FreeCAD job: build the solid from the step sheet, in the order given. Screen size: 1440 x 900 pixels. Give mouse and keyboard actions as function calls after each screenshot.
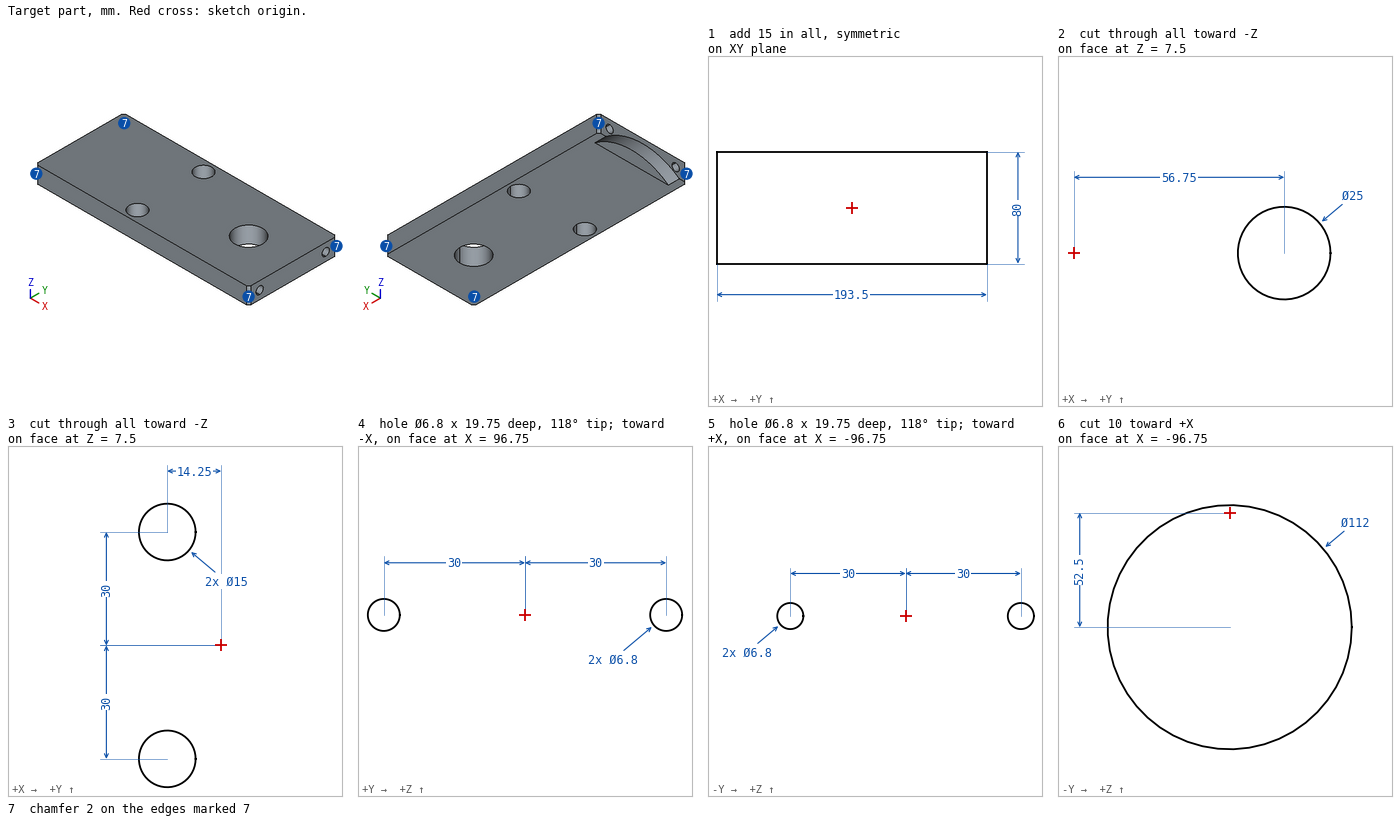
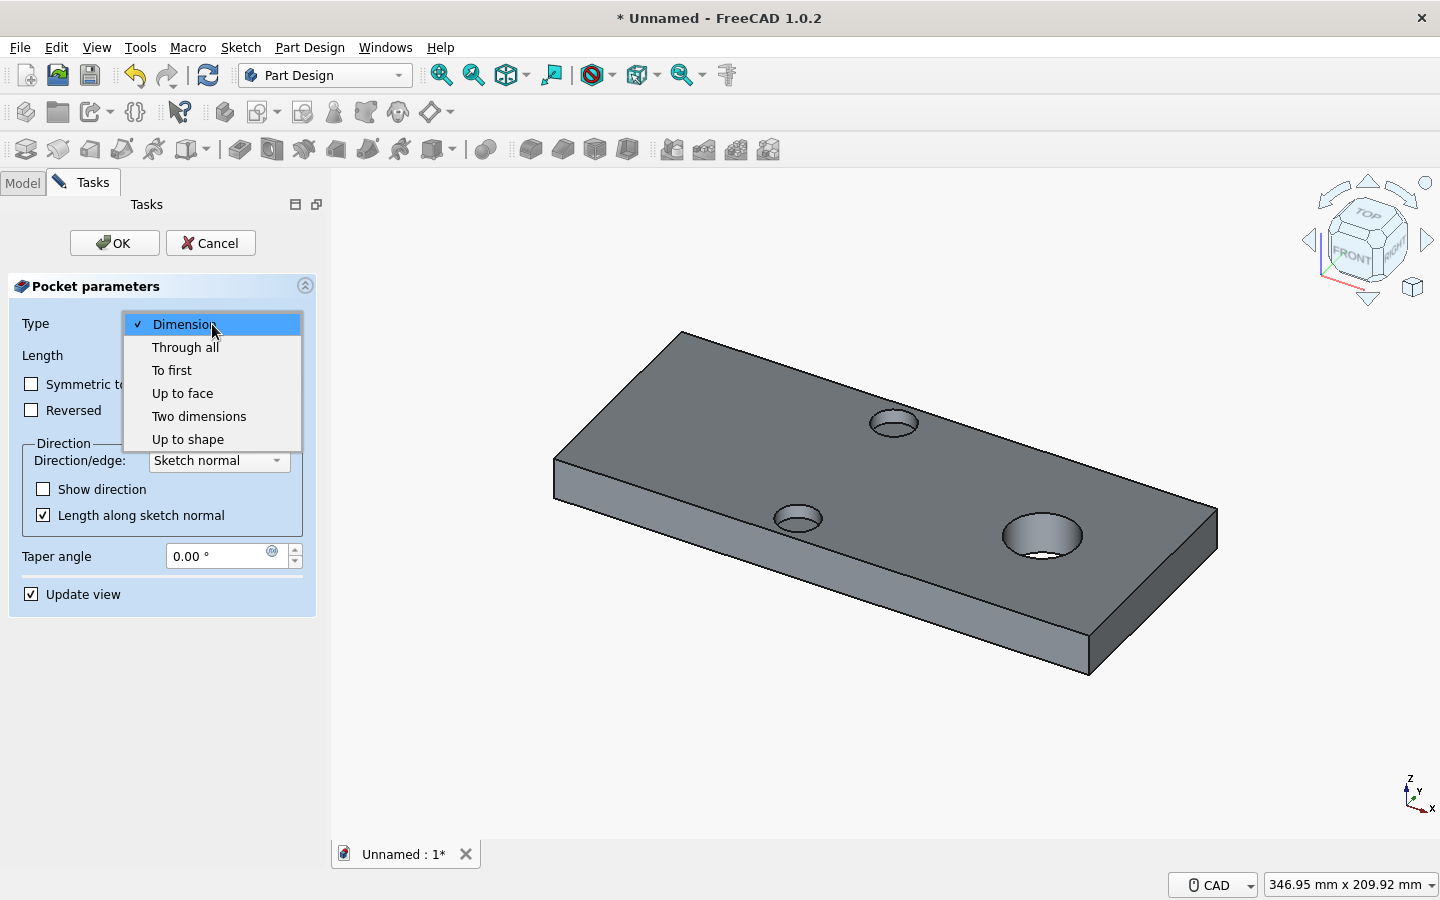
click(212, 348)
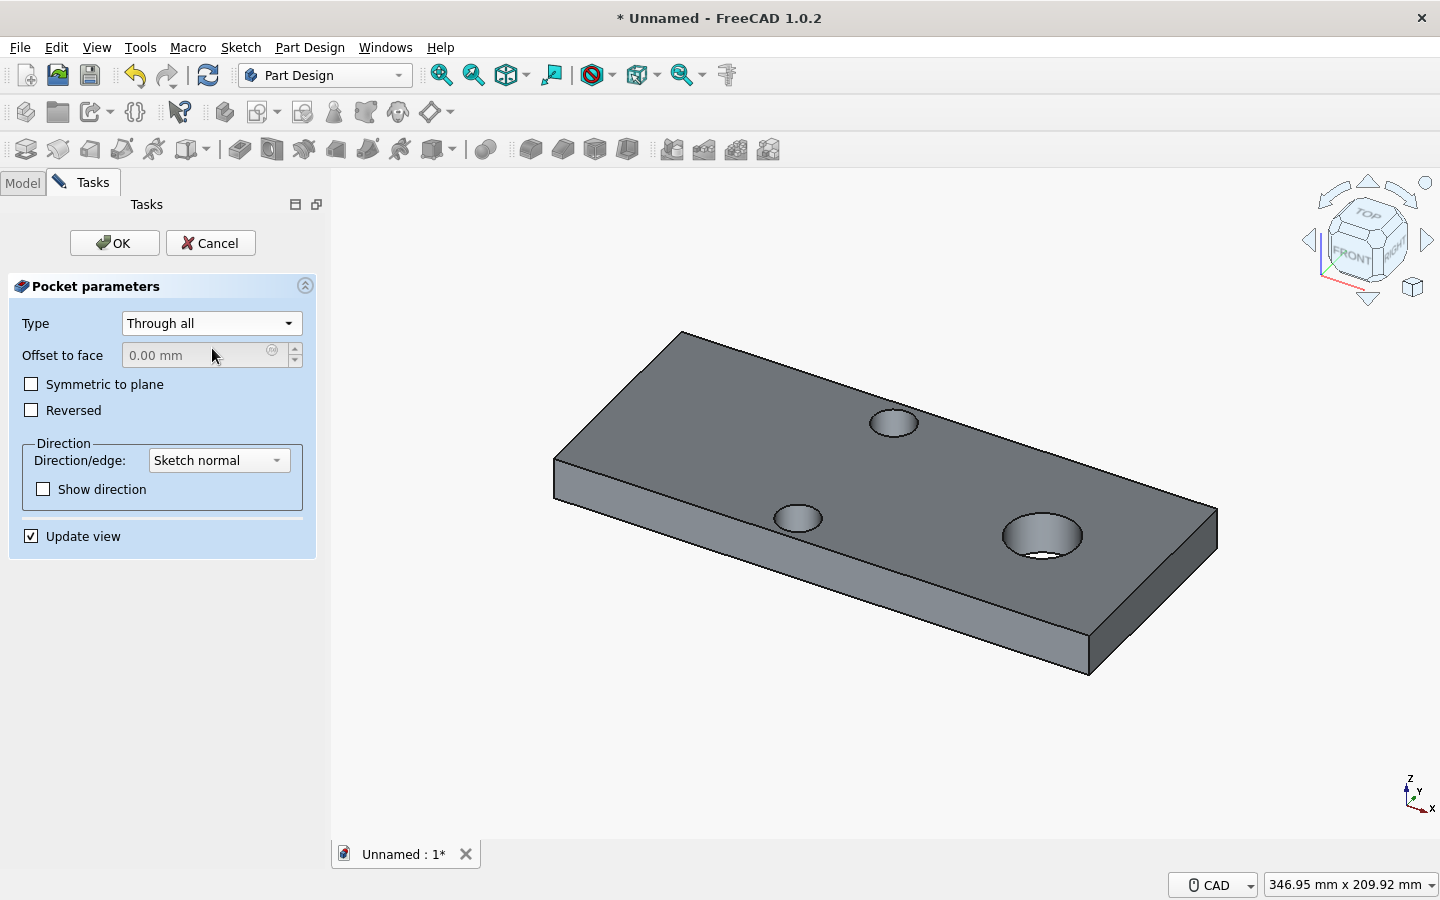
click(115, 243)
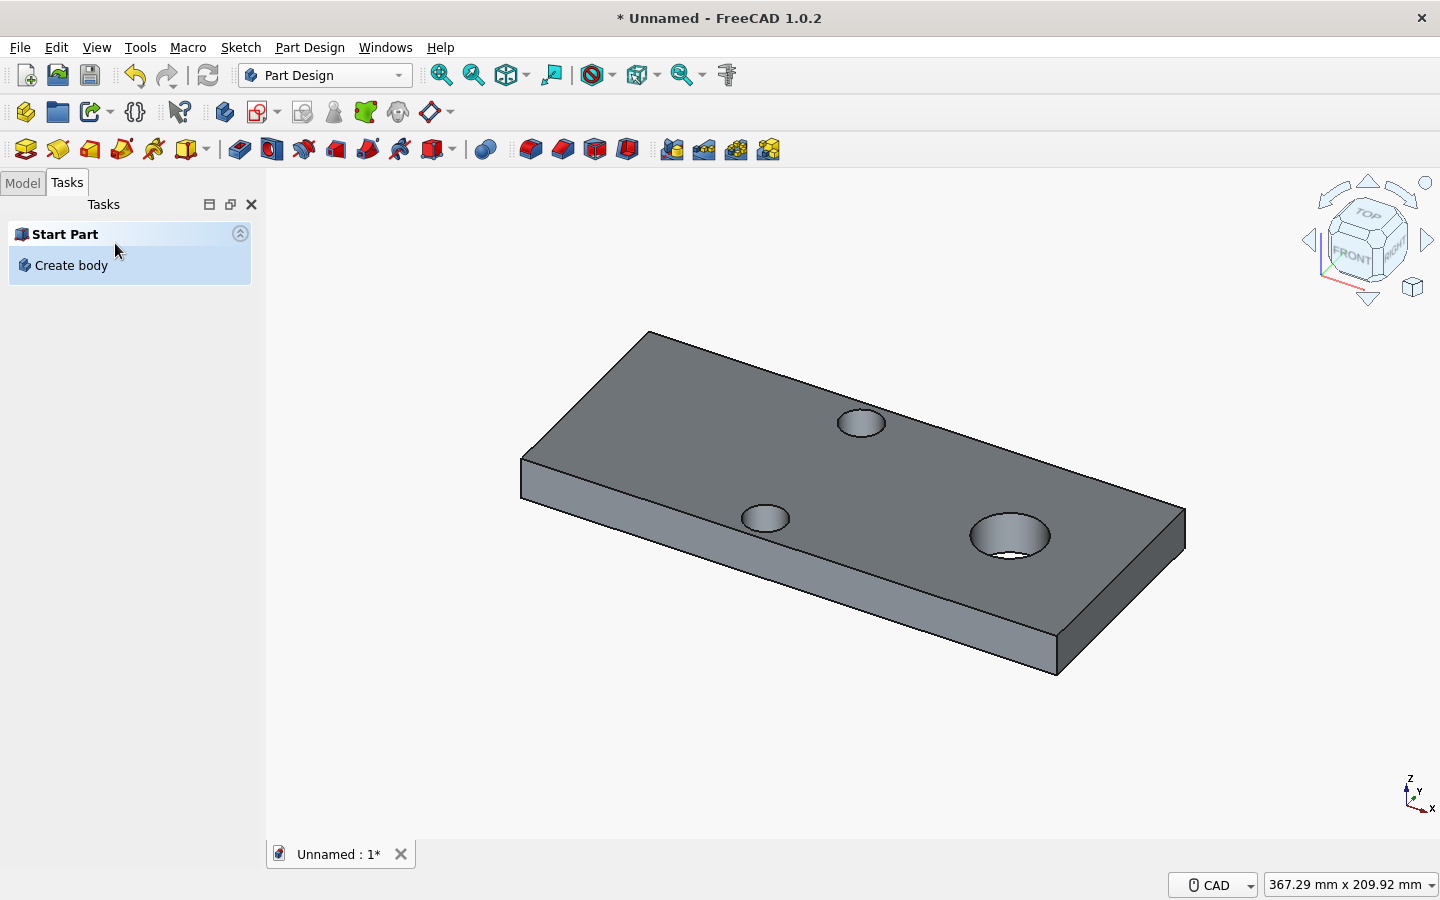
click(1157, 555)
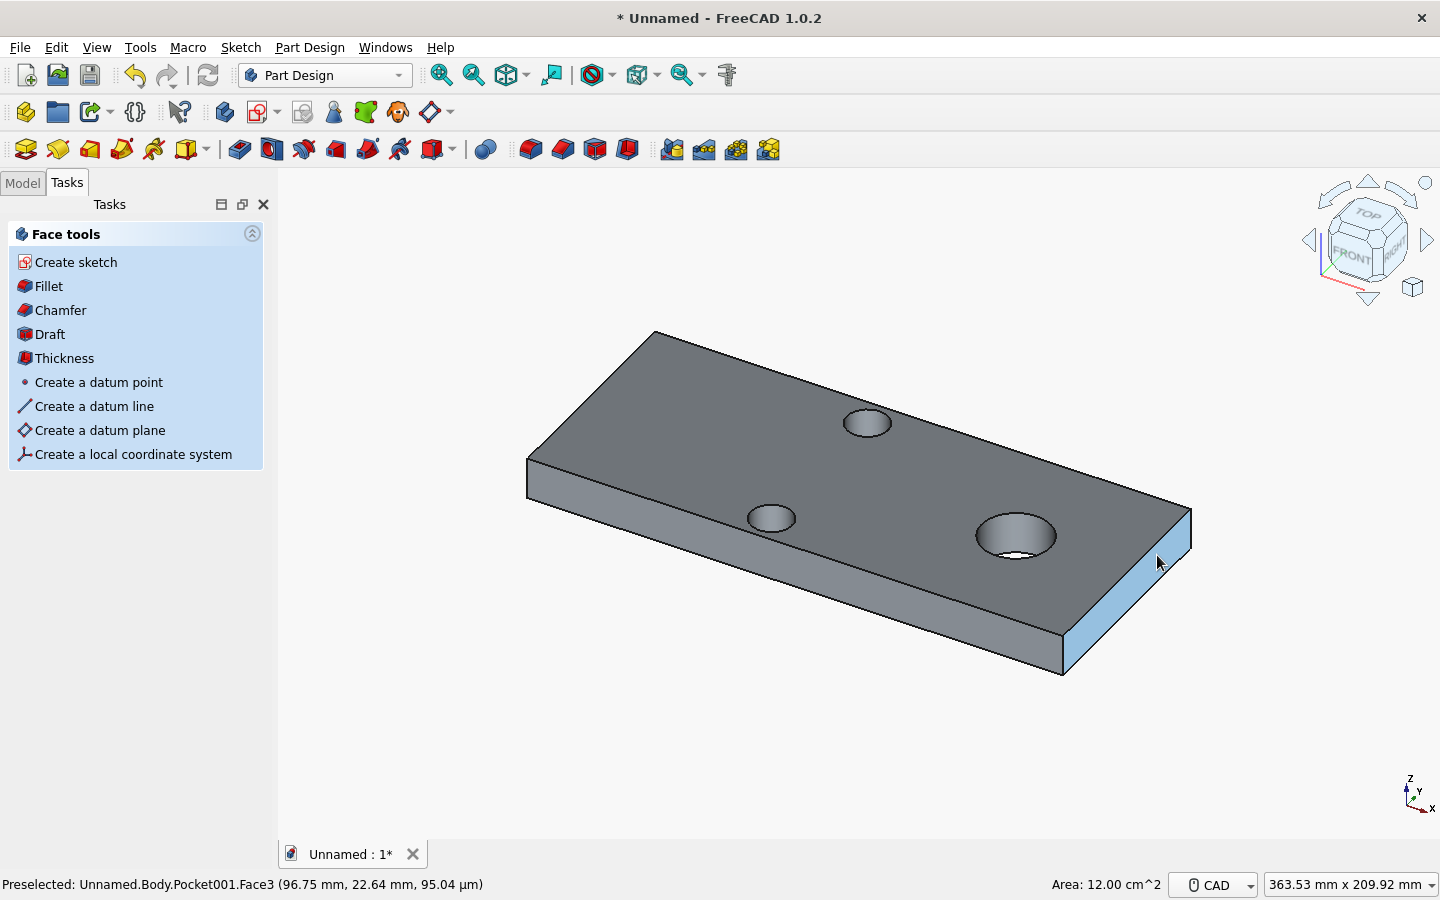
click(258, 112)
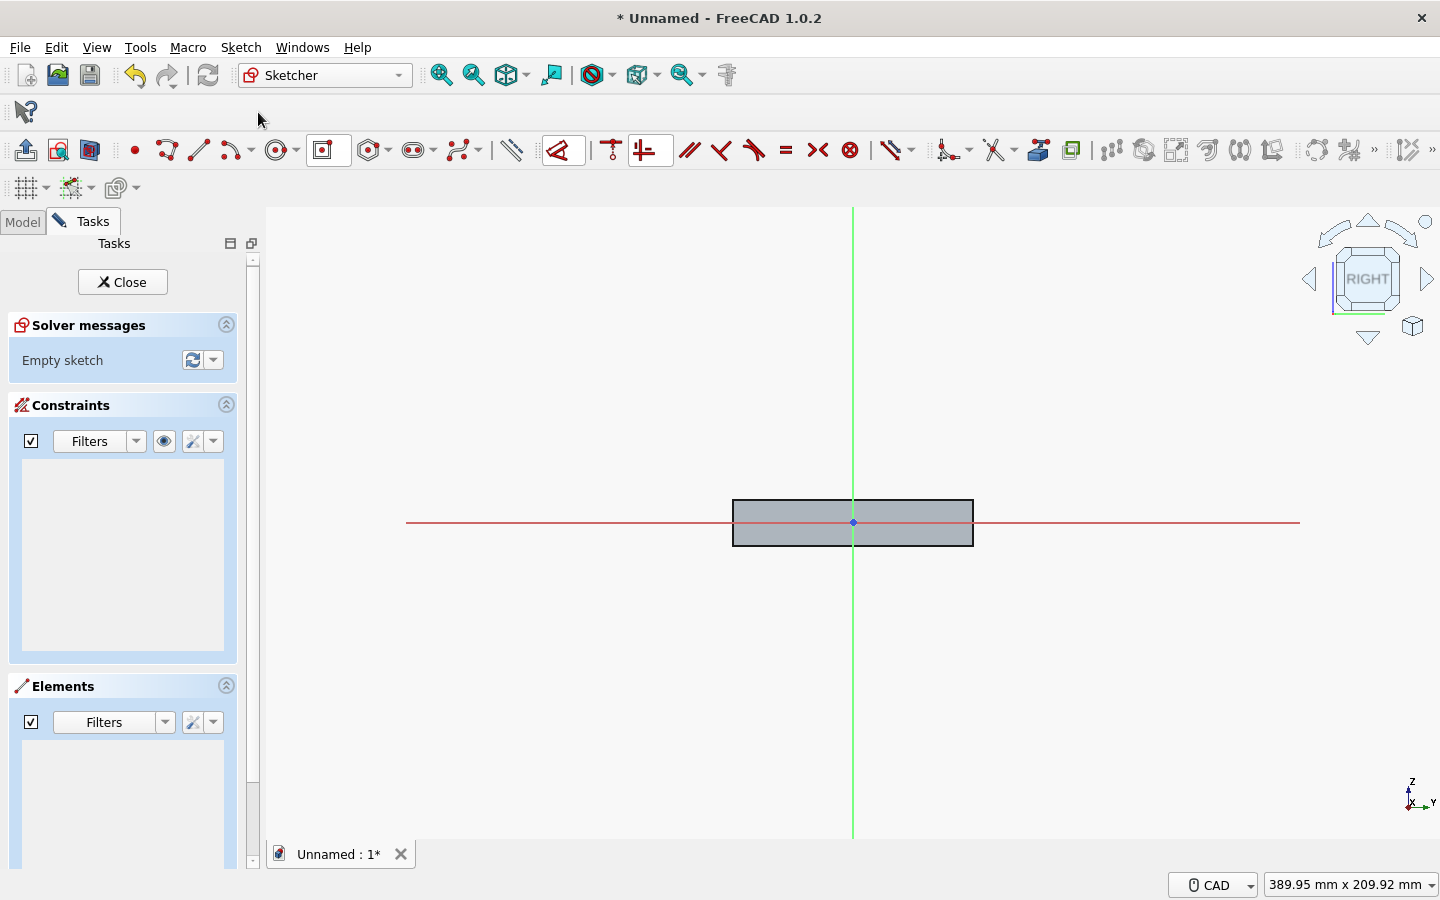
scroll(883, 523, up, 6)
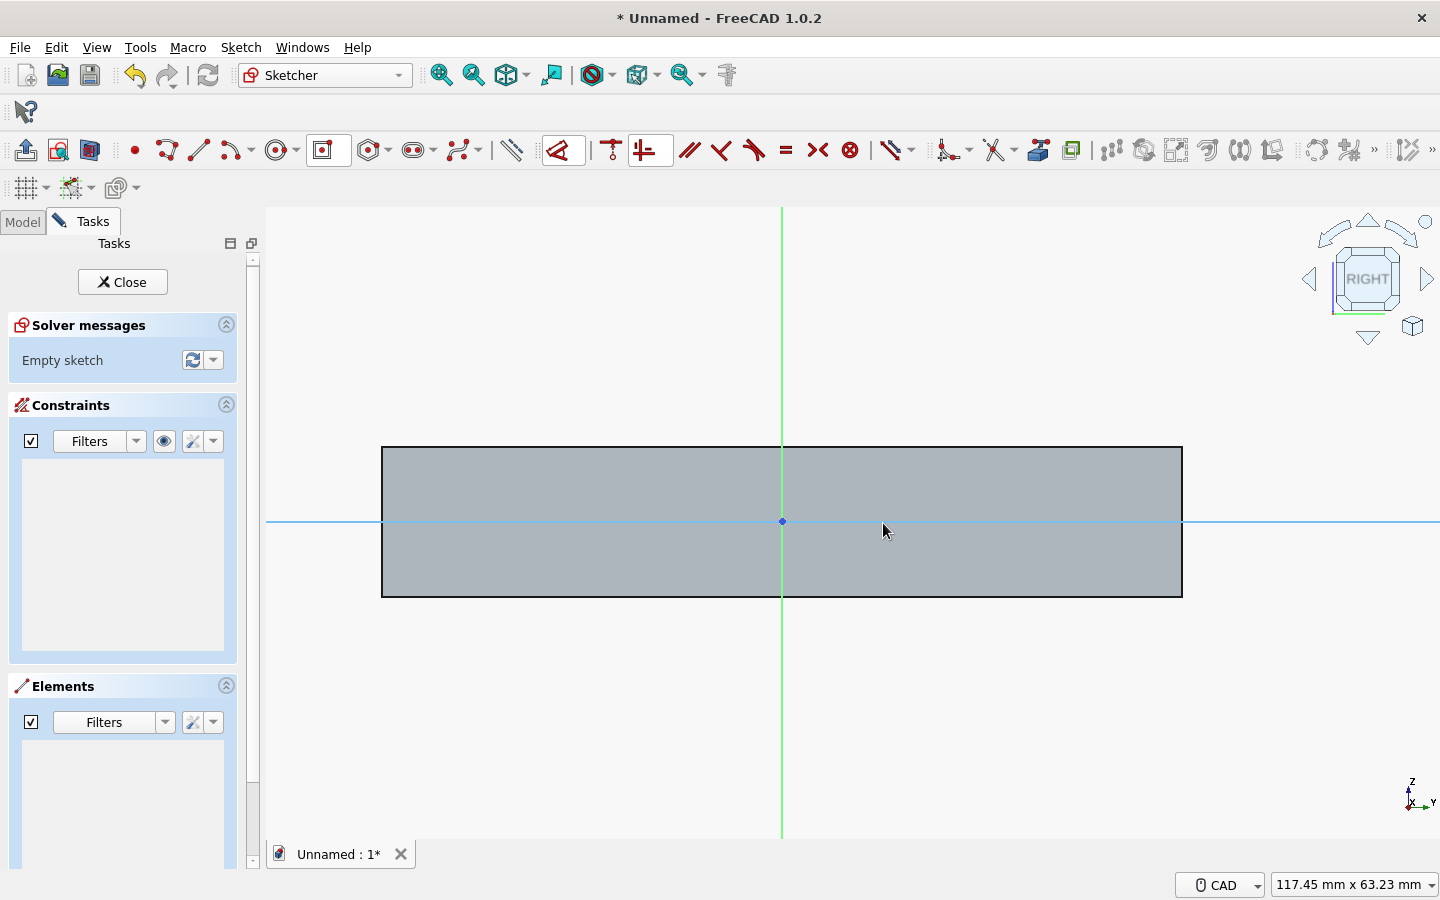
click(276, 150)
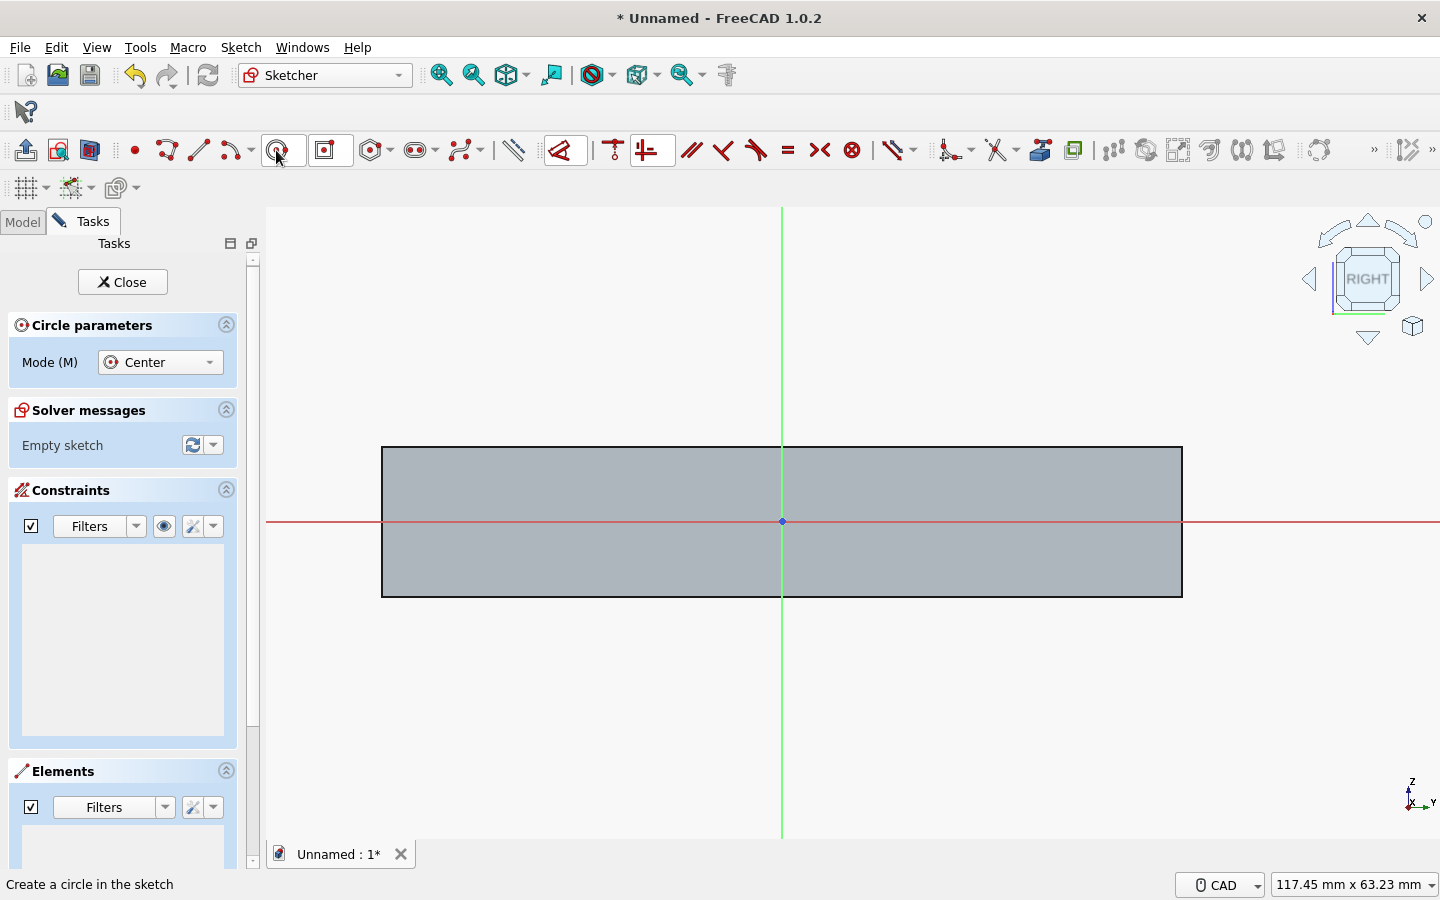
click(1082, 522)
move(1106, 498)